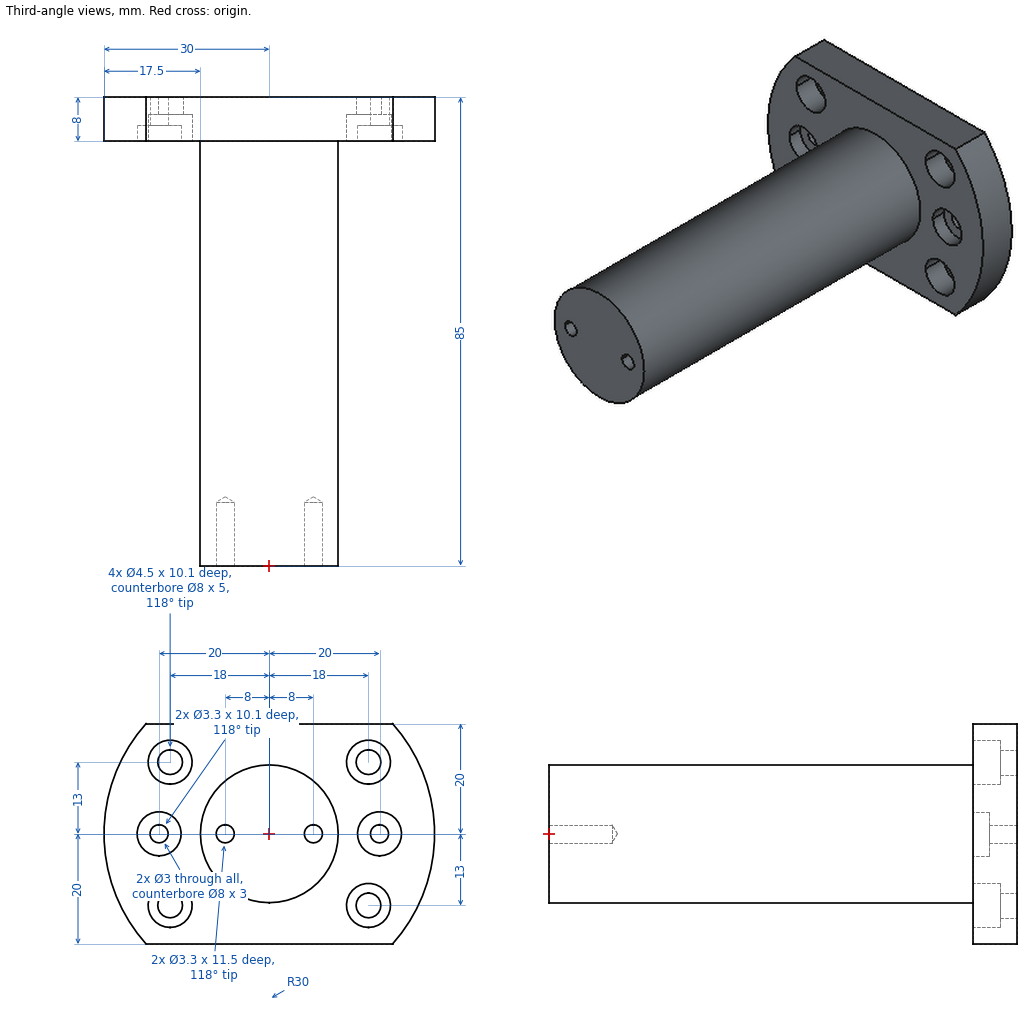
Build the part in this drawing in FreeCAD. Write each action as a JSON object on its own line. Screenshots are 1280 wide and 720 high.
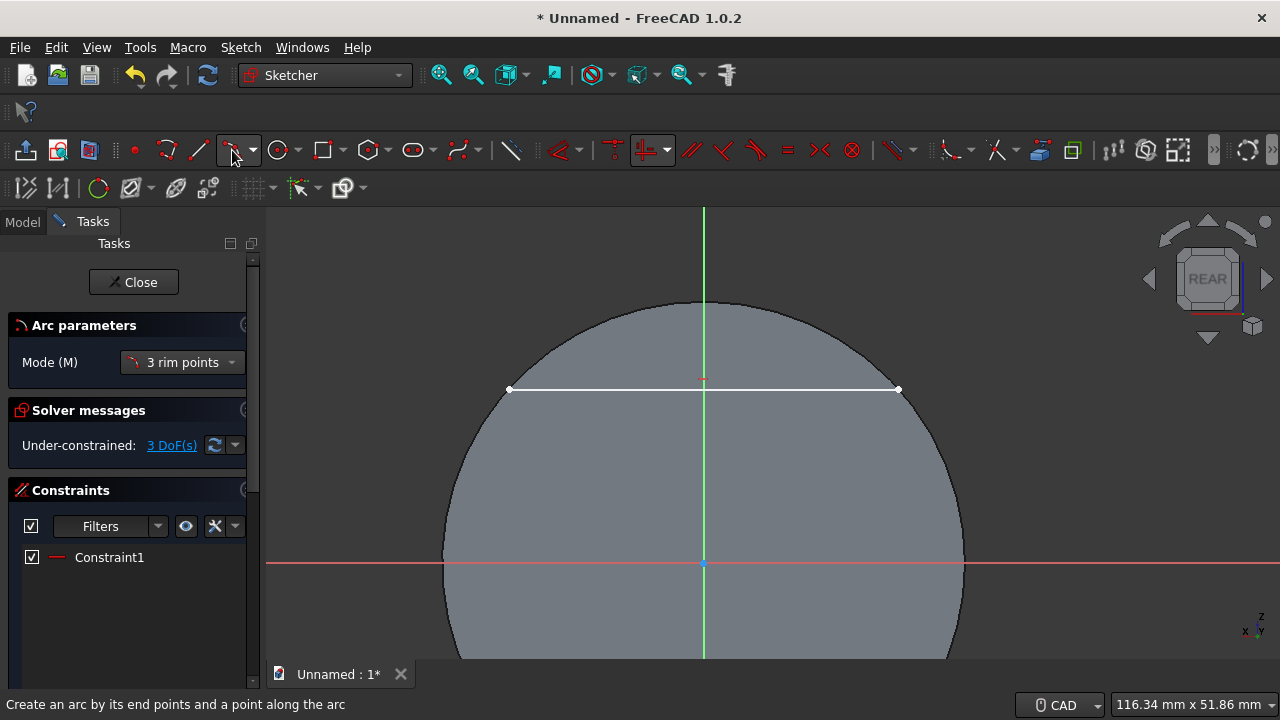
{"action": "left_click", "coordinate": [898, 390]}
{"action": "left_click", "coordinate": [509, 390]}
{"action": "left_click", "coordinate": [747, 305]}
{"action": "key", "text": "Escape"}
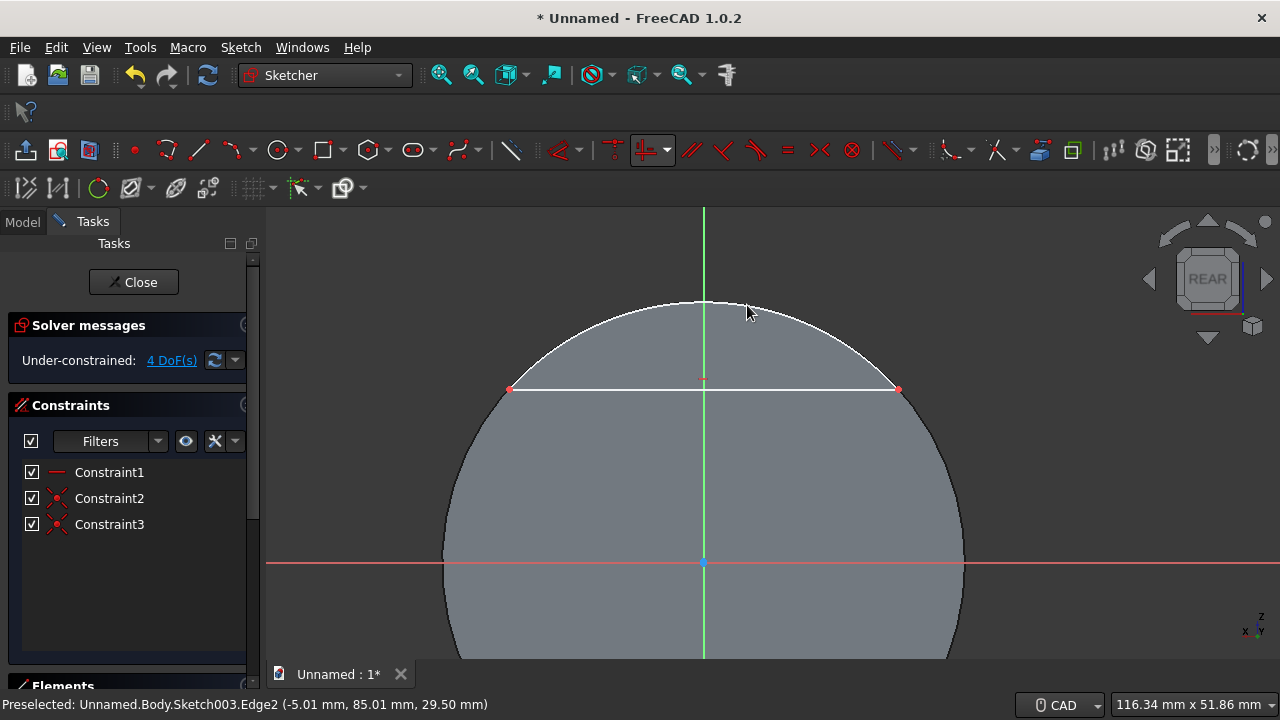
{"action": "left_click_drag", "start_coordinate": [694, 552], "coordinate": [714, 573]}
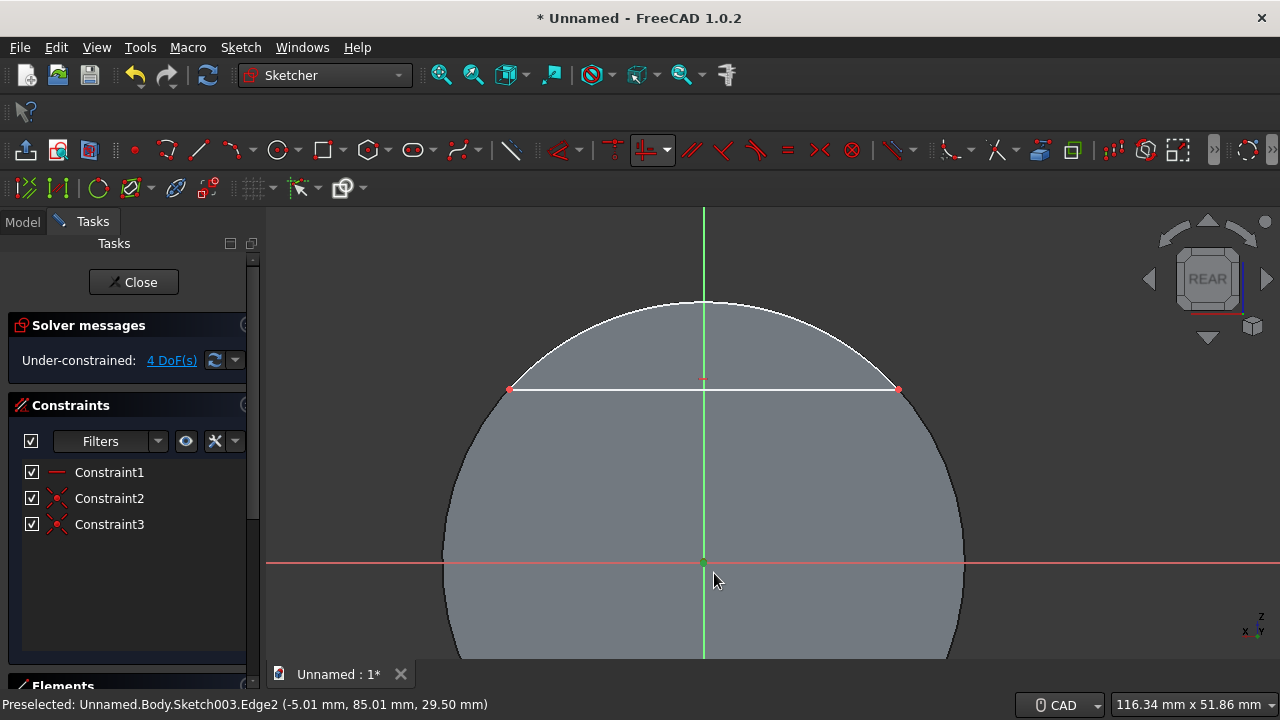
{"action": "left_click", "coordinate": [614, 150]}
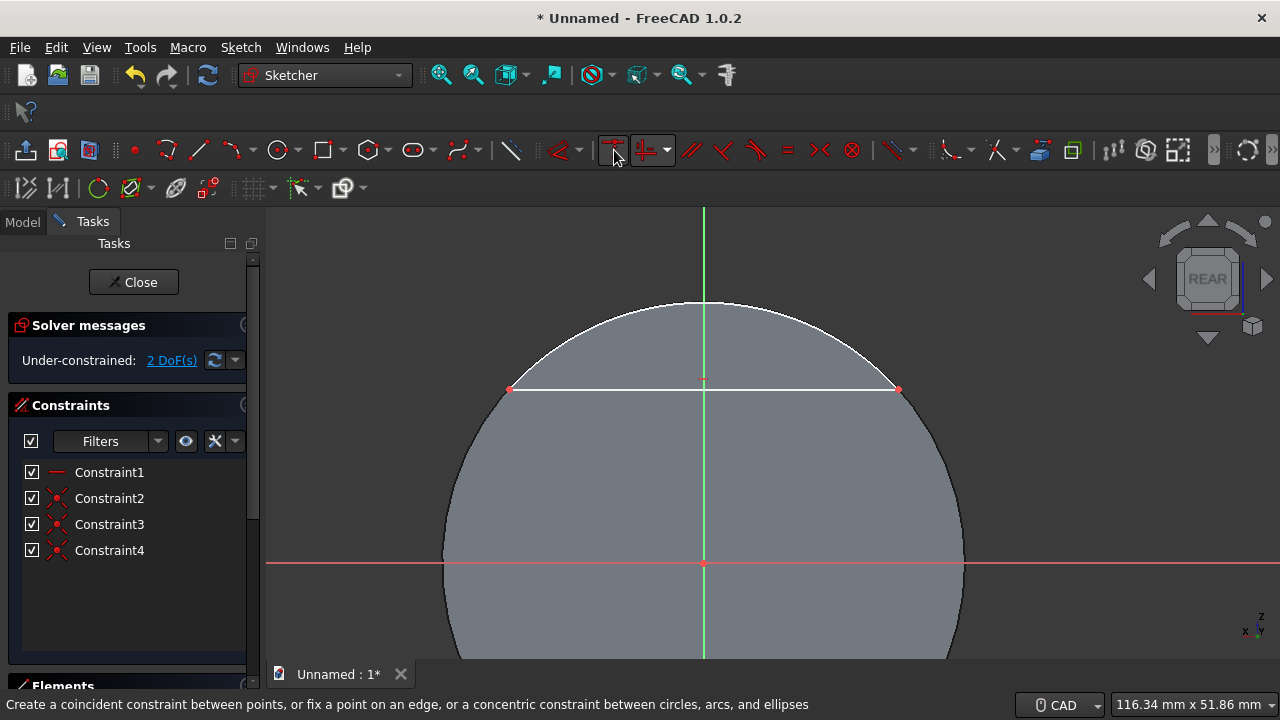
{"action": "left_click", "coordinate": [558, 150]}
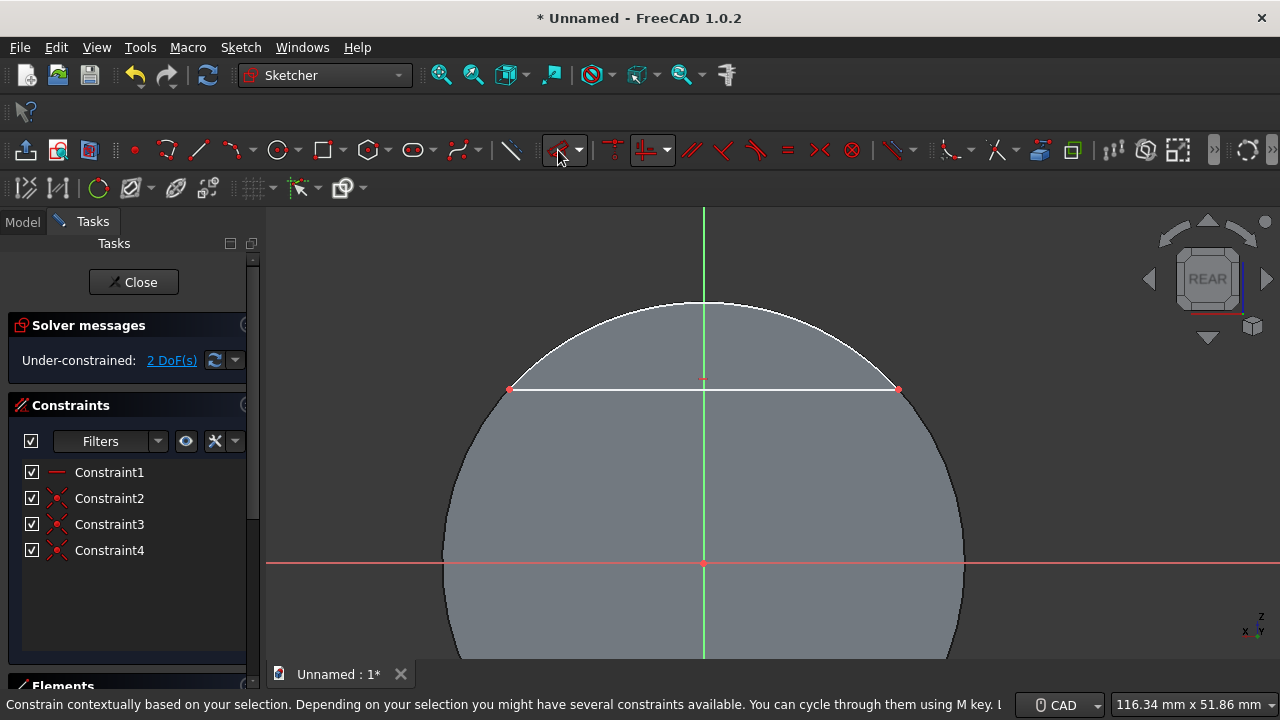
{"action": "left_click", "coordinate": [790, 317]}
{"action": "left_click", "coordinate": [801, 287]}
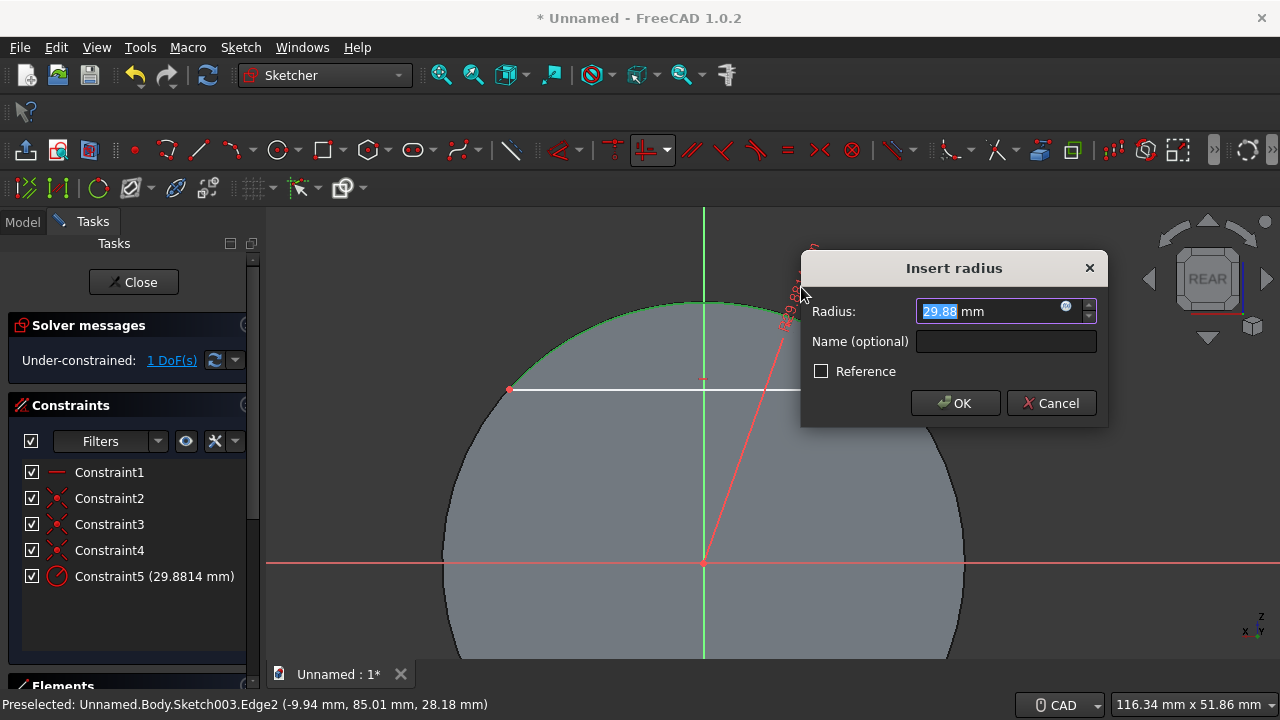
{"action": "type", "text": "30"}
{"action": "key", "text": "Return"}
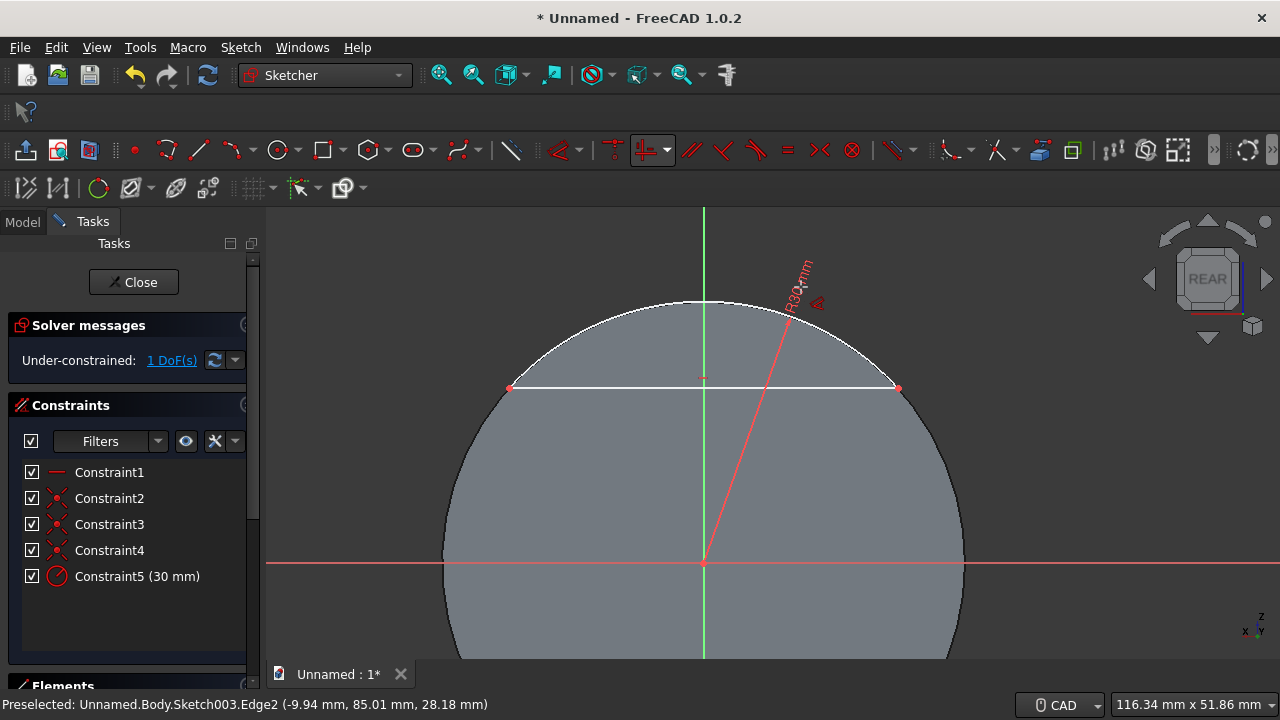
{"action": "left_click", "coordinate": [509, 388]}
{"action": "left_click", "coordinate": [475, 476]}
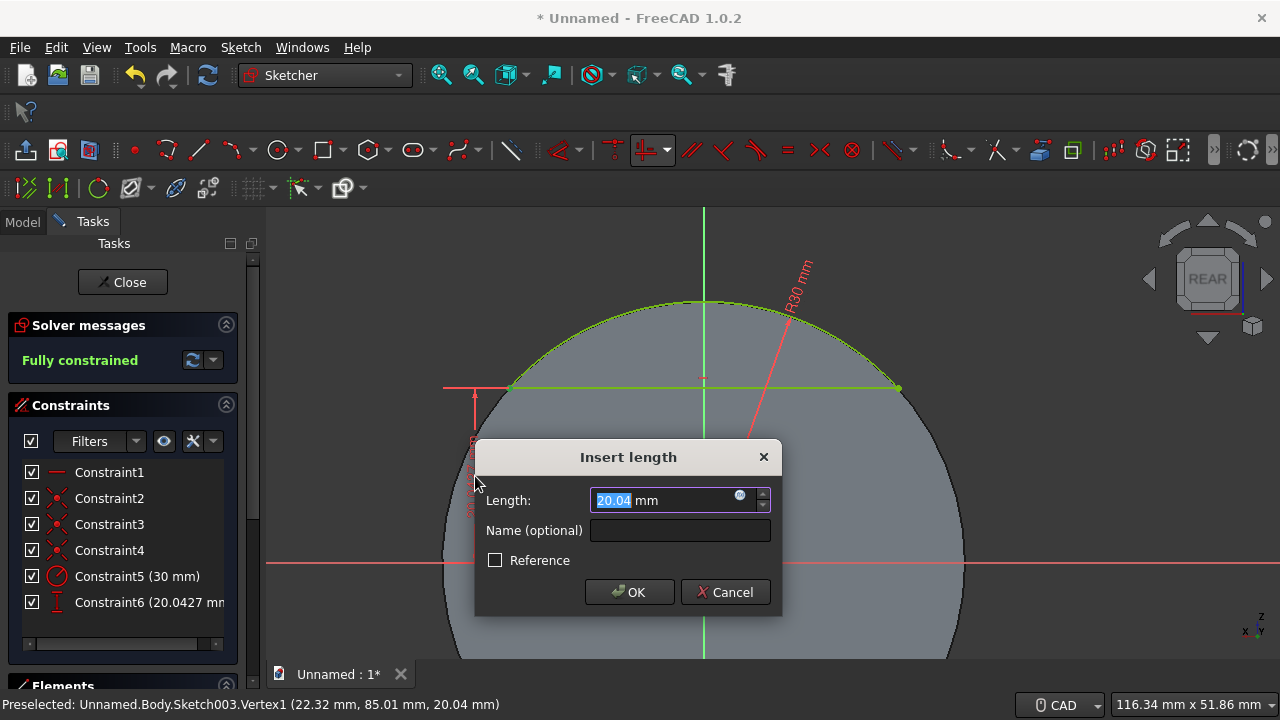
{"action": "type", "text": "20"}
{"action": "key", "text": "Return"}
{"action": "key", "text": "Escape"}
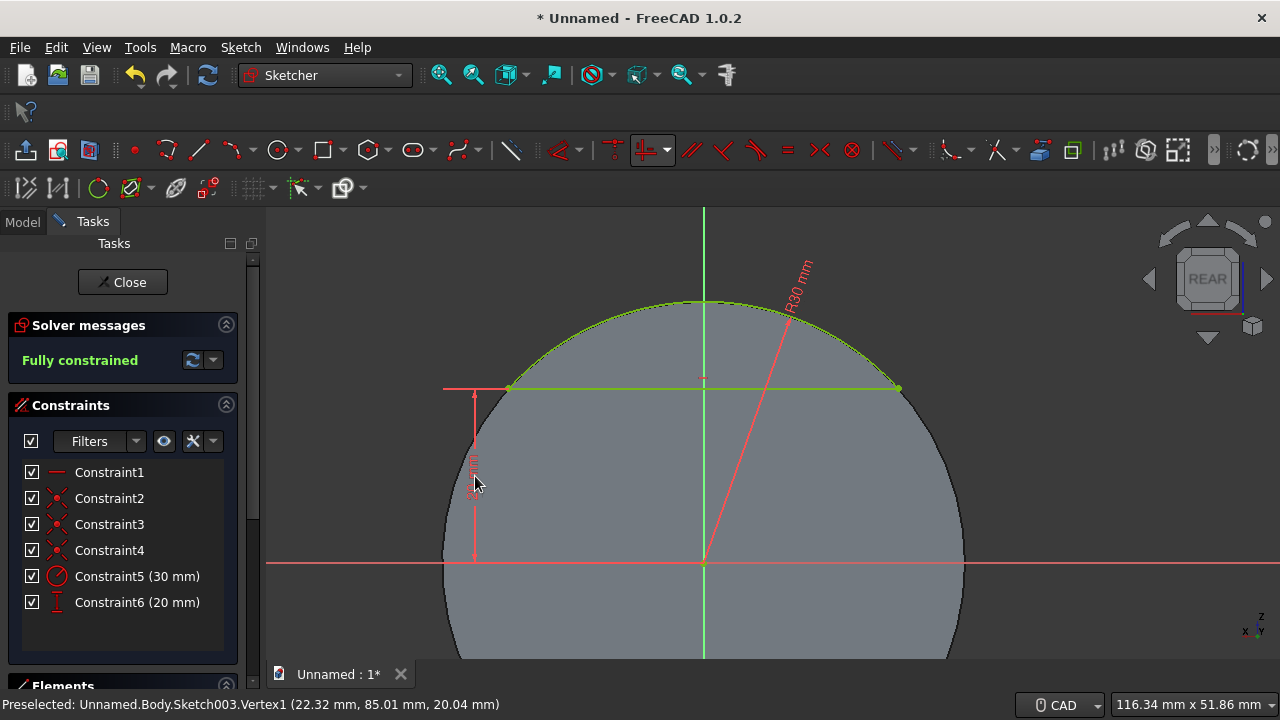
{"action": "left_click", "coordinate": [123, 282]}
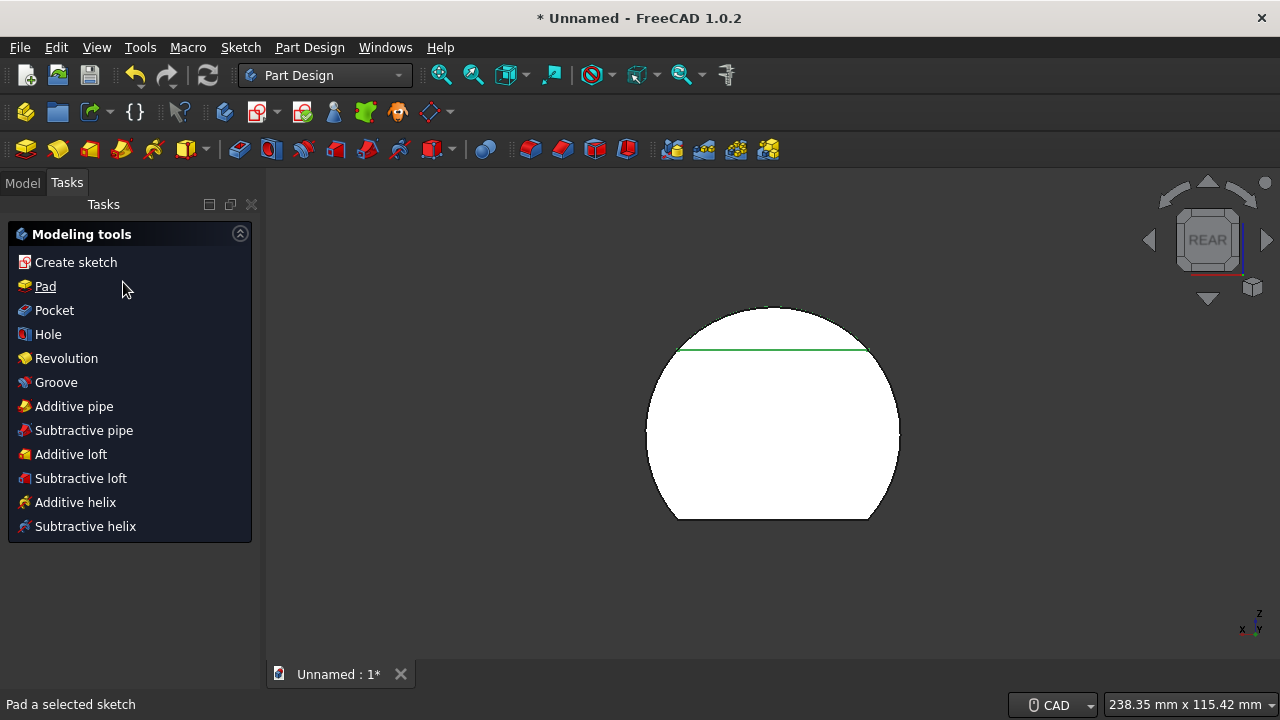
{"action": "left_click", "coordinate": [240, 150]}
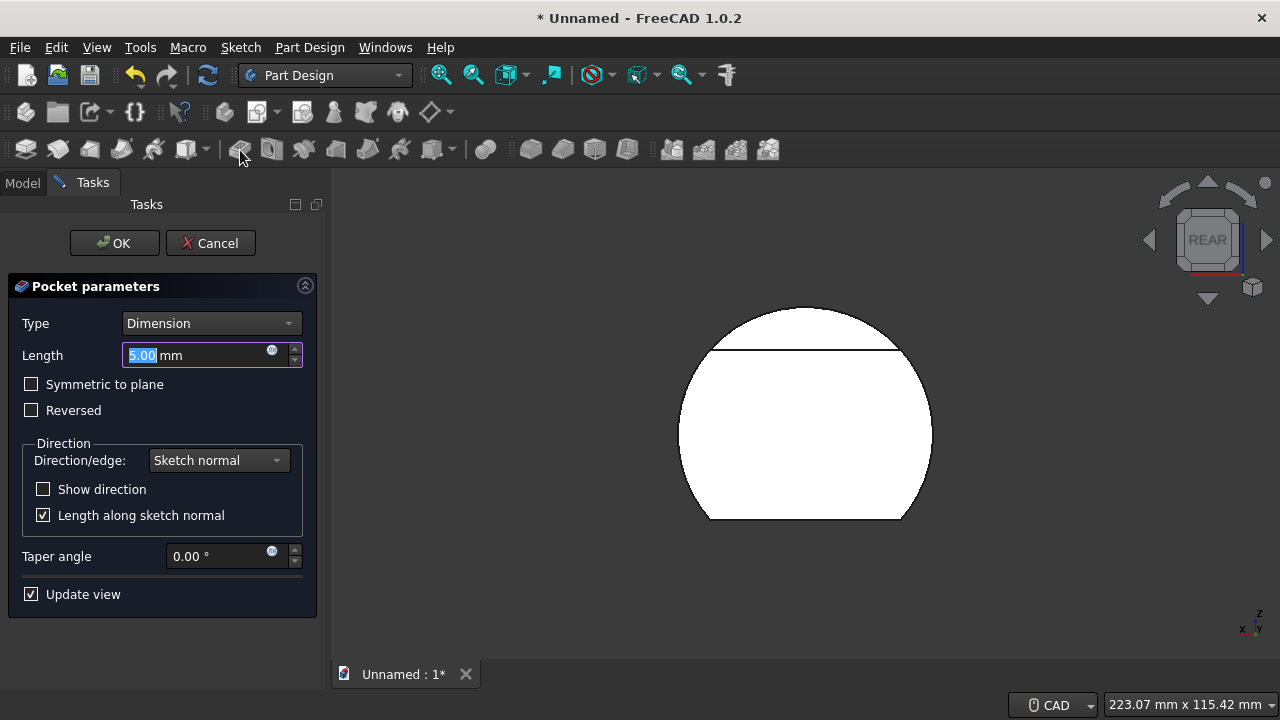
{"action": "left_click", "coordinate": [212, 324]}